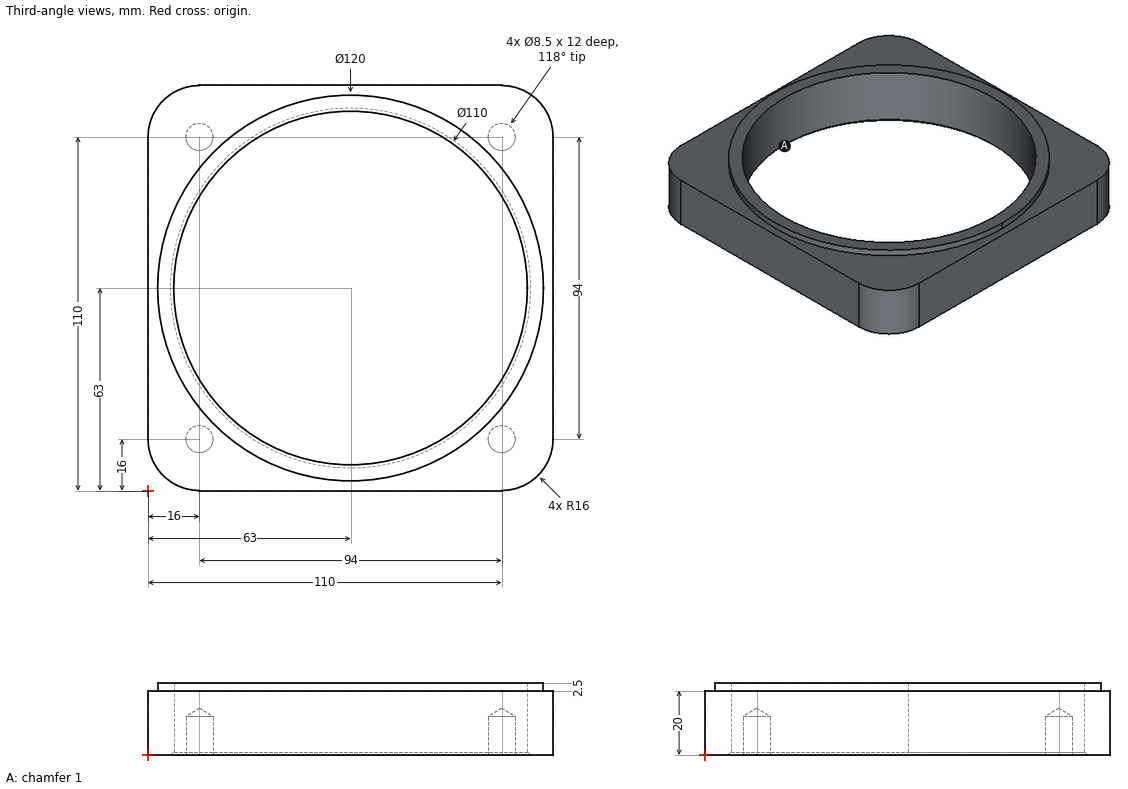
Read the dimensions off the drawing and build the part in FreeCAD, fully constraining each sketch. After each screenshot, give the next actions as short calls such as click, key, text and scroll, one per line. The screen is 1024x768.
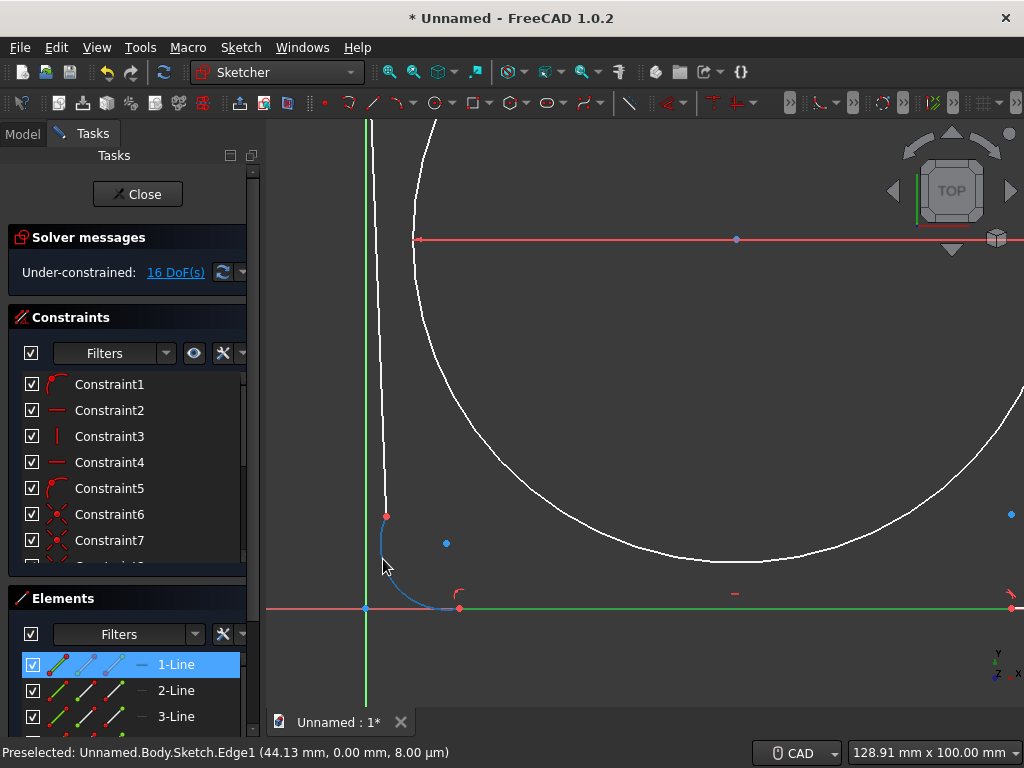
click(382, 559)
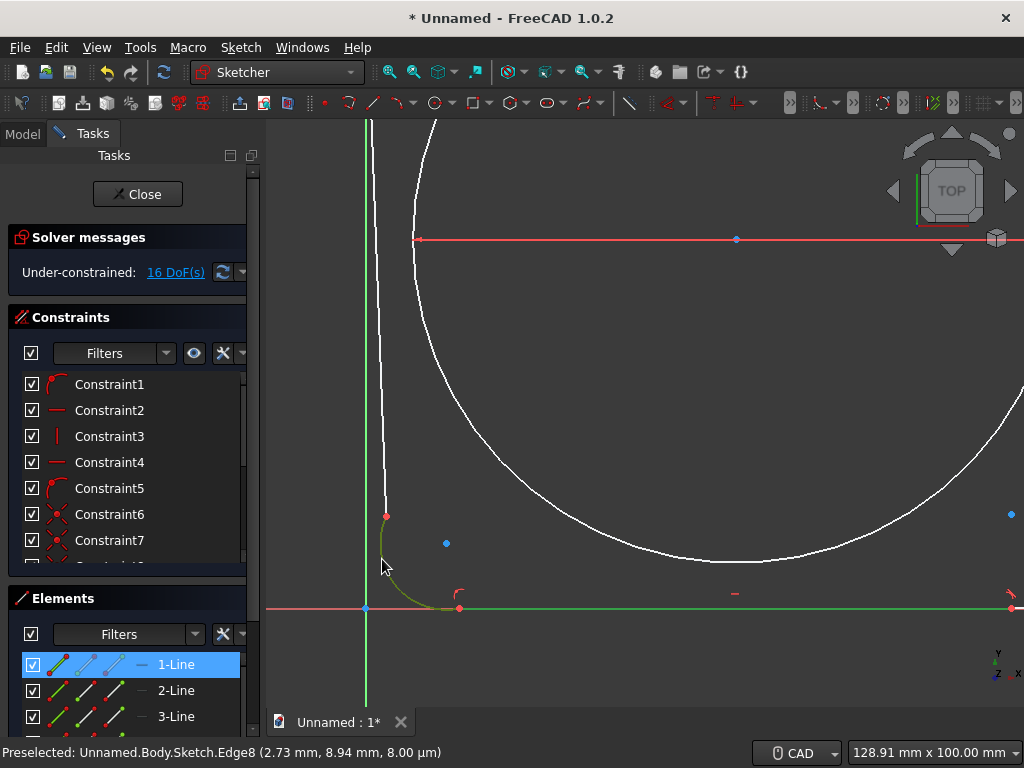
key(t)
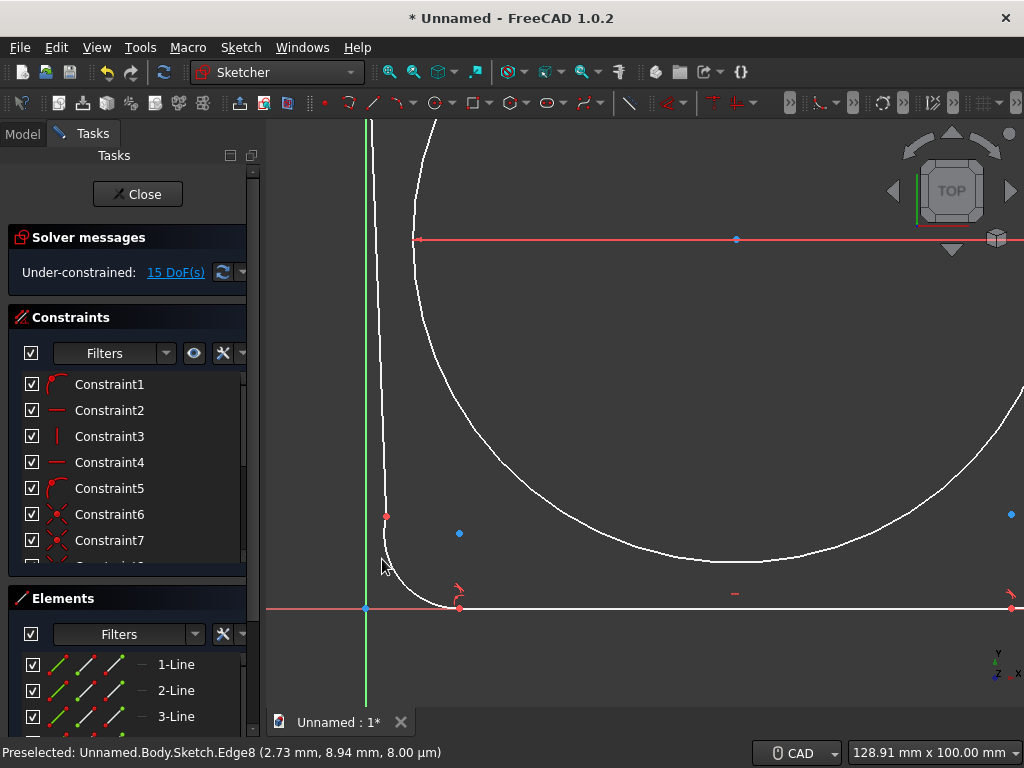
scroll(382, 626, down, 3)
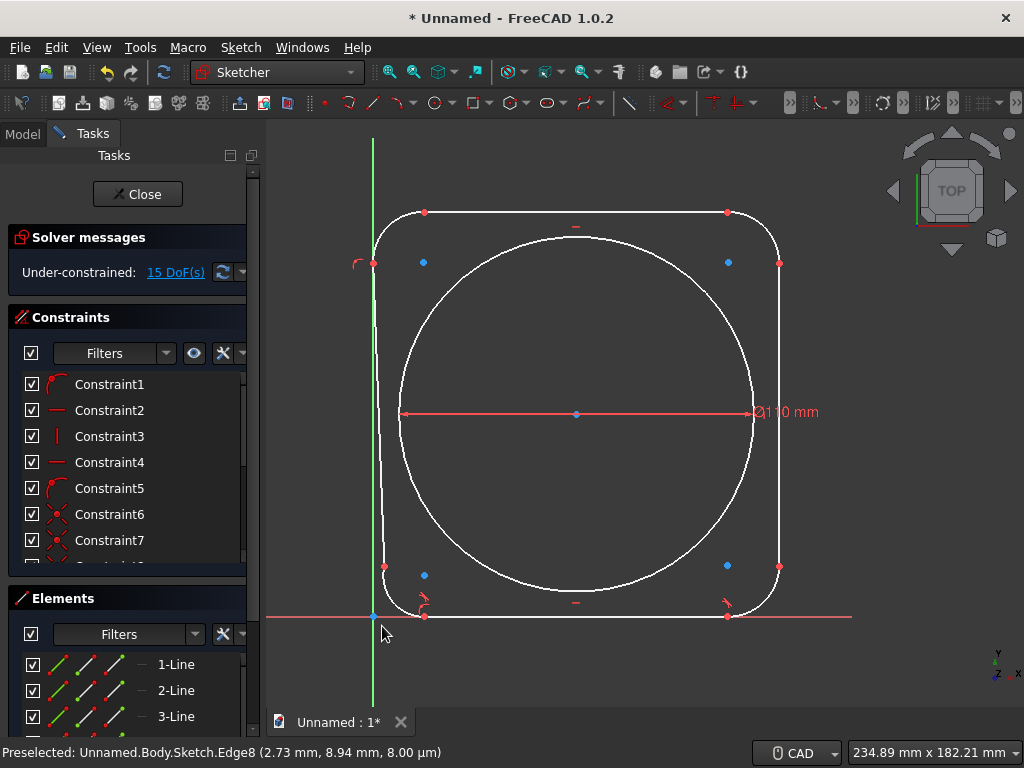
click(779, 475)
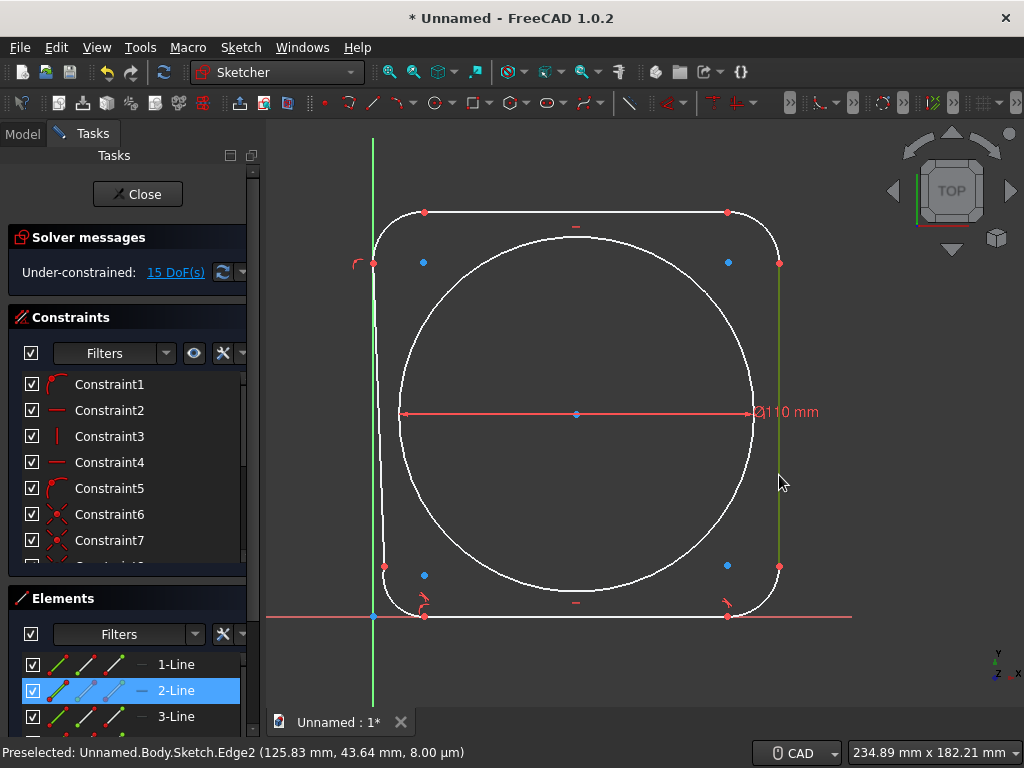
click(773, 589)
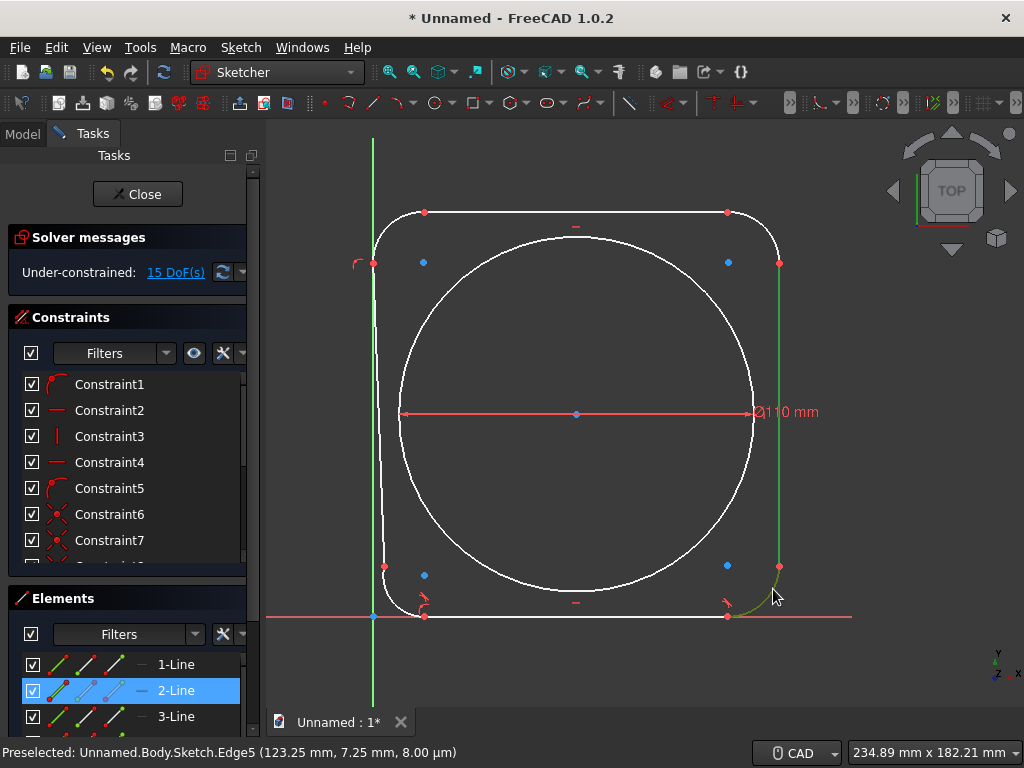
key(t)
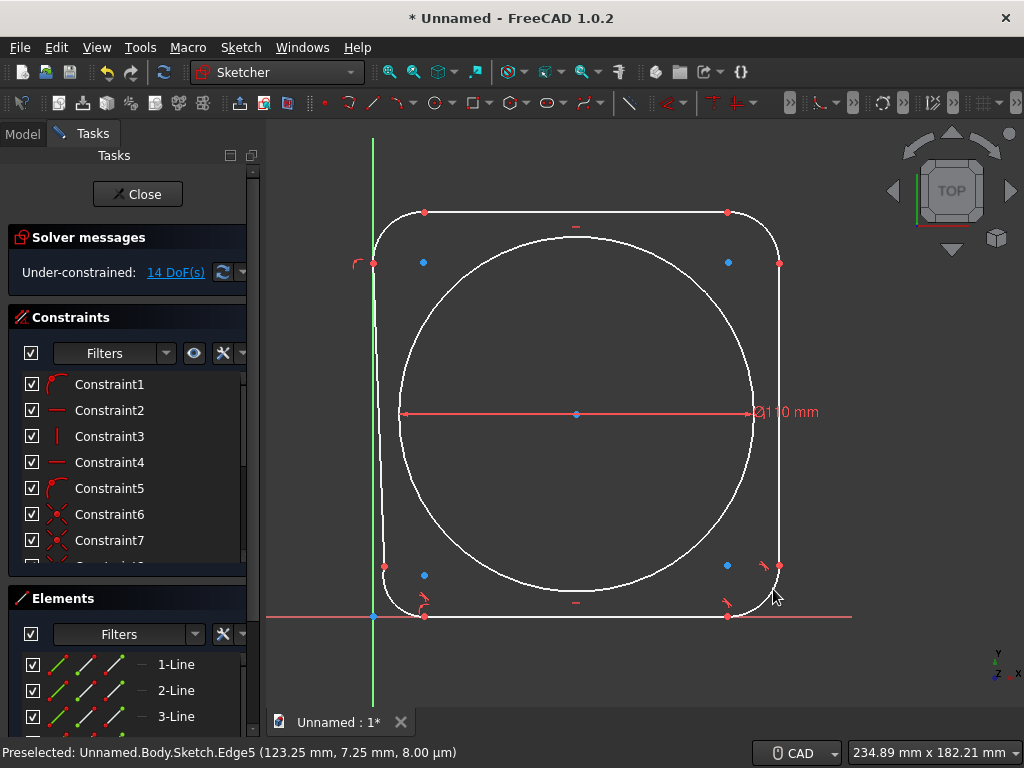
click(779, 475)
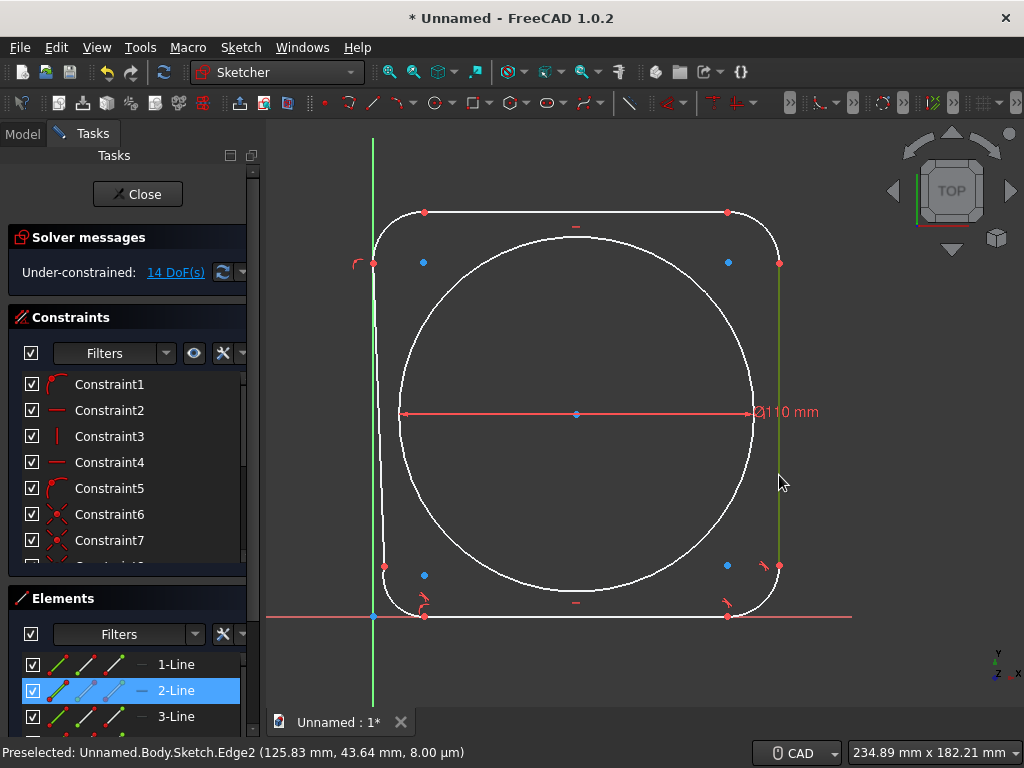
click(774, 240)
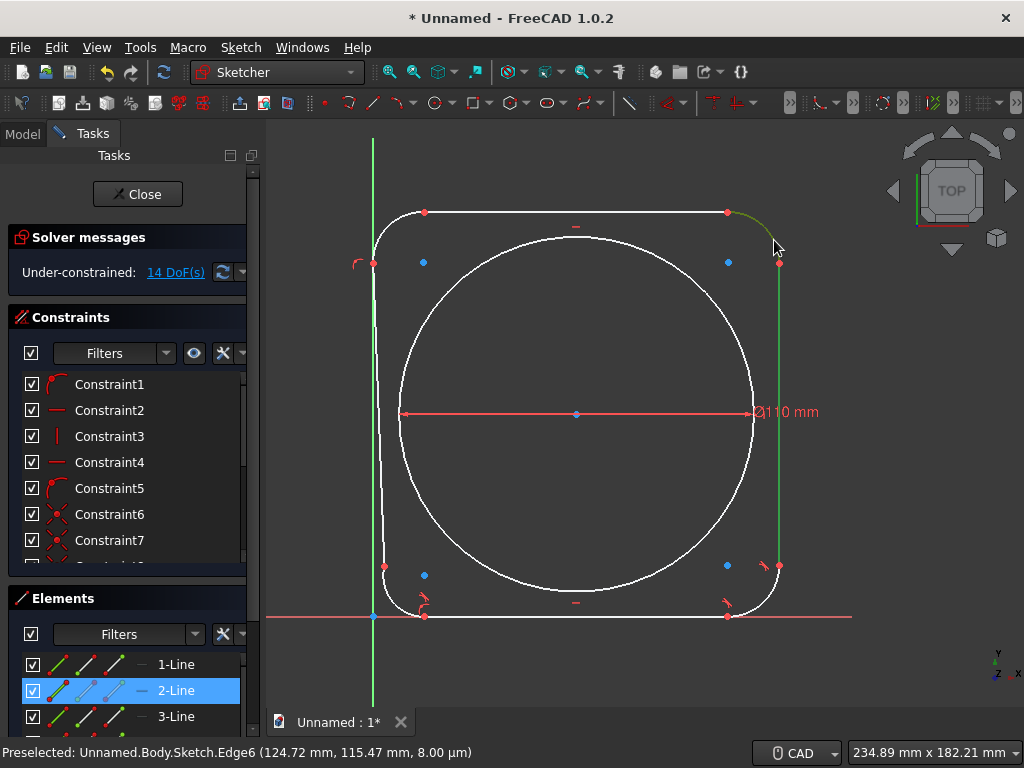
key(t)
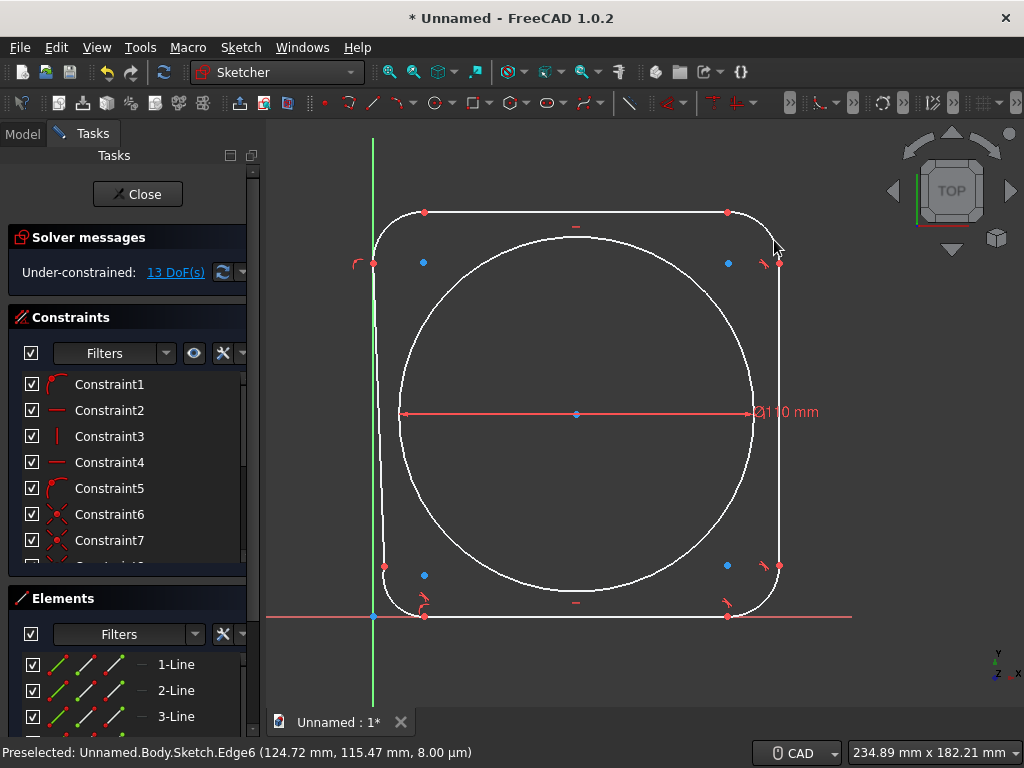
click(637, 212)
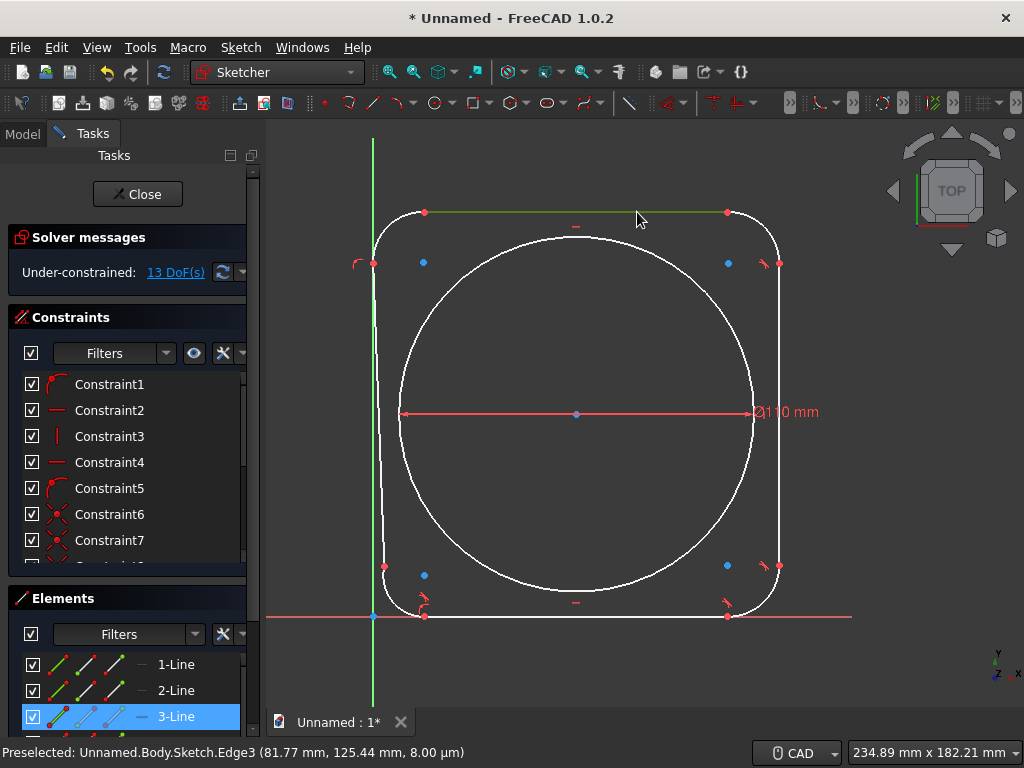
click(774, 240)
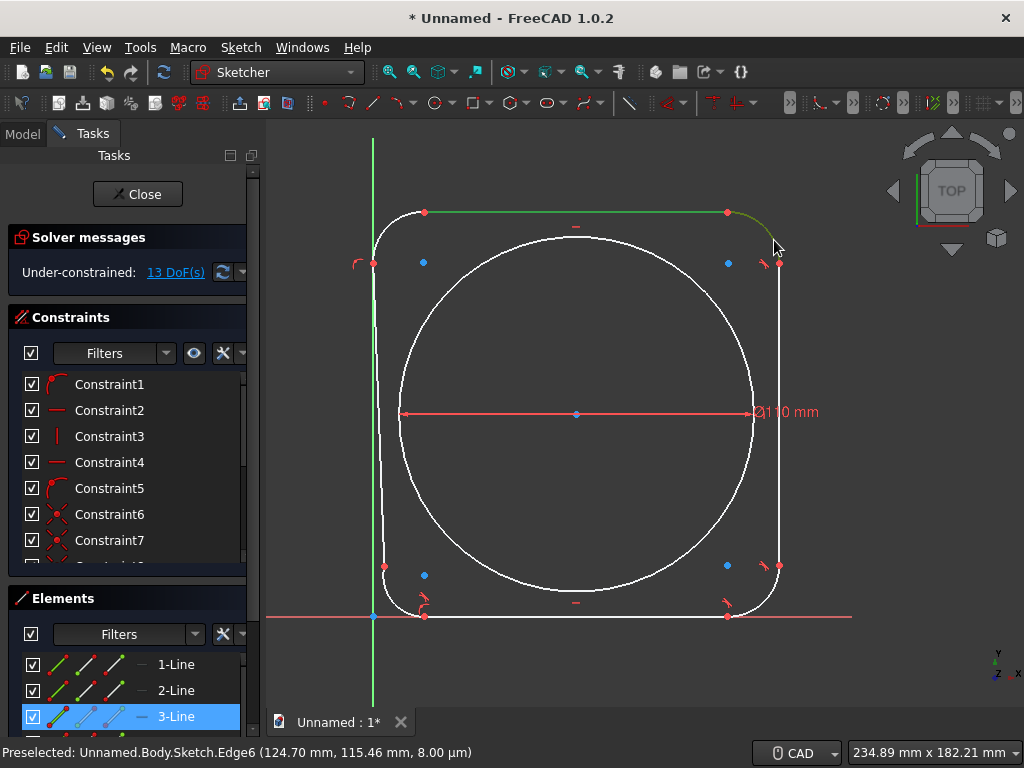
key(t)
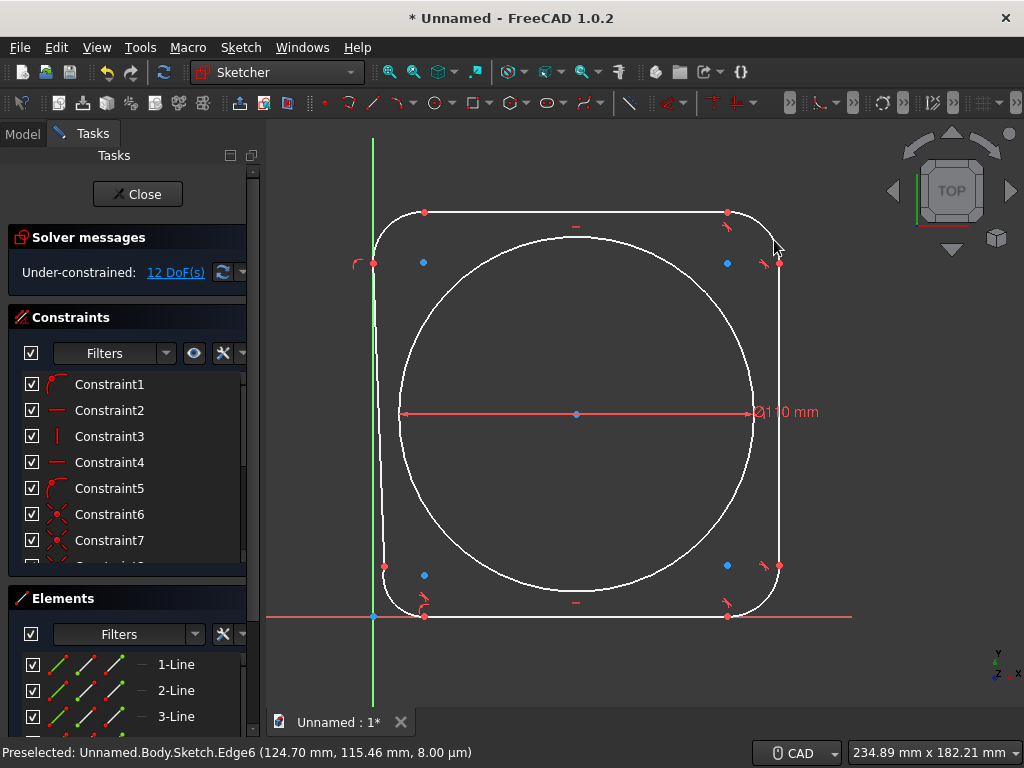
click(637, 212)